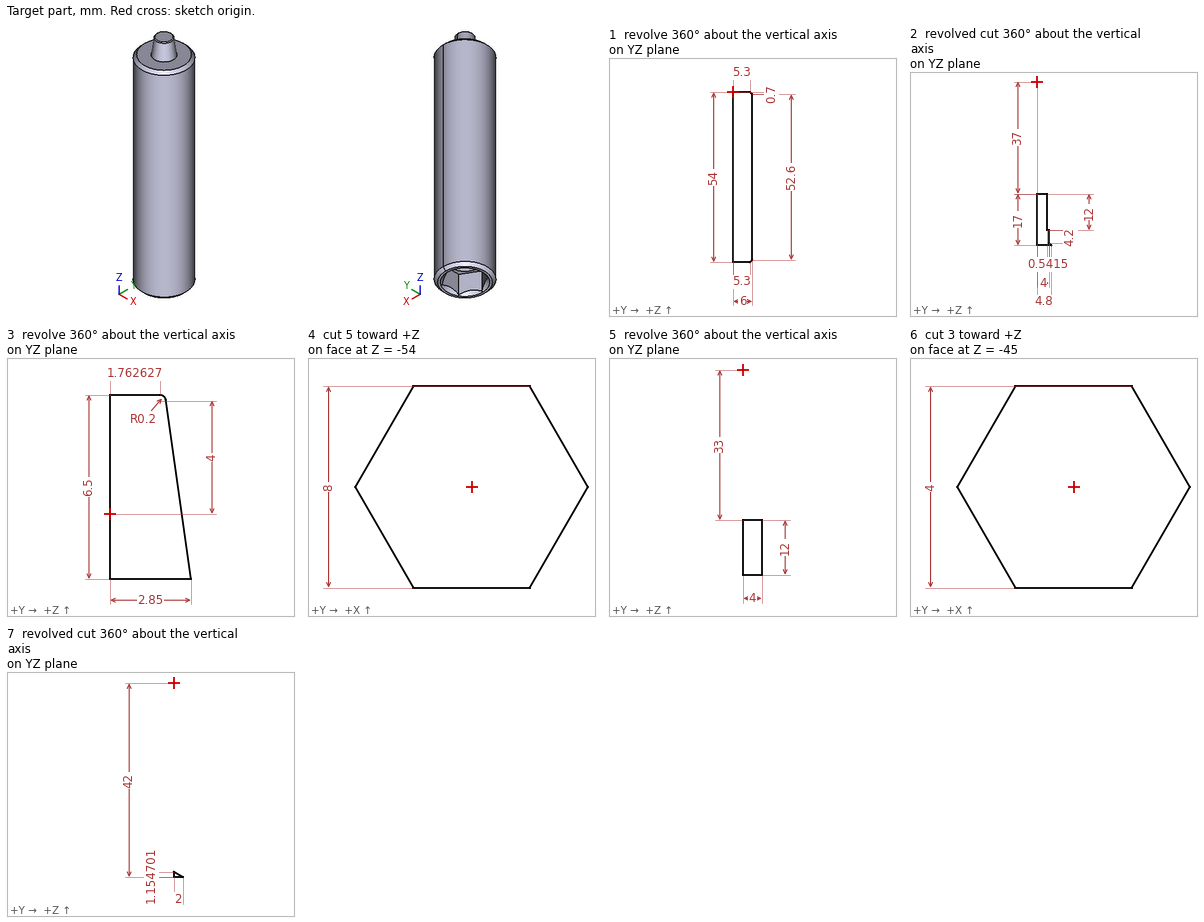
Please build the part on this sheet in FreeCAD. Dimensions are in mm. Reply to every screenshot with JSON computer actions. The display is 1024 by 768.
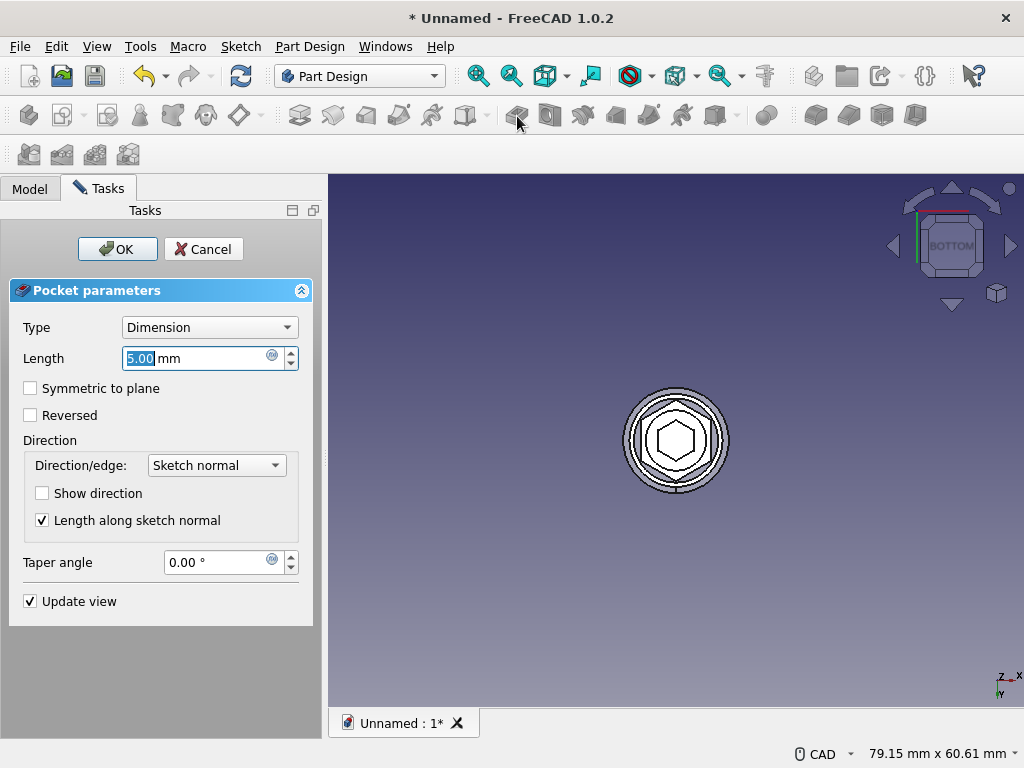
{"action": "type", "text": "3"}
{"action": "key", "text": "Tab"}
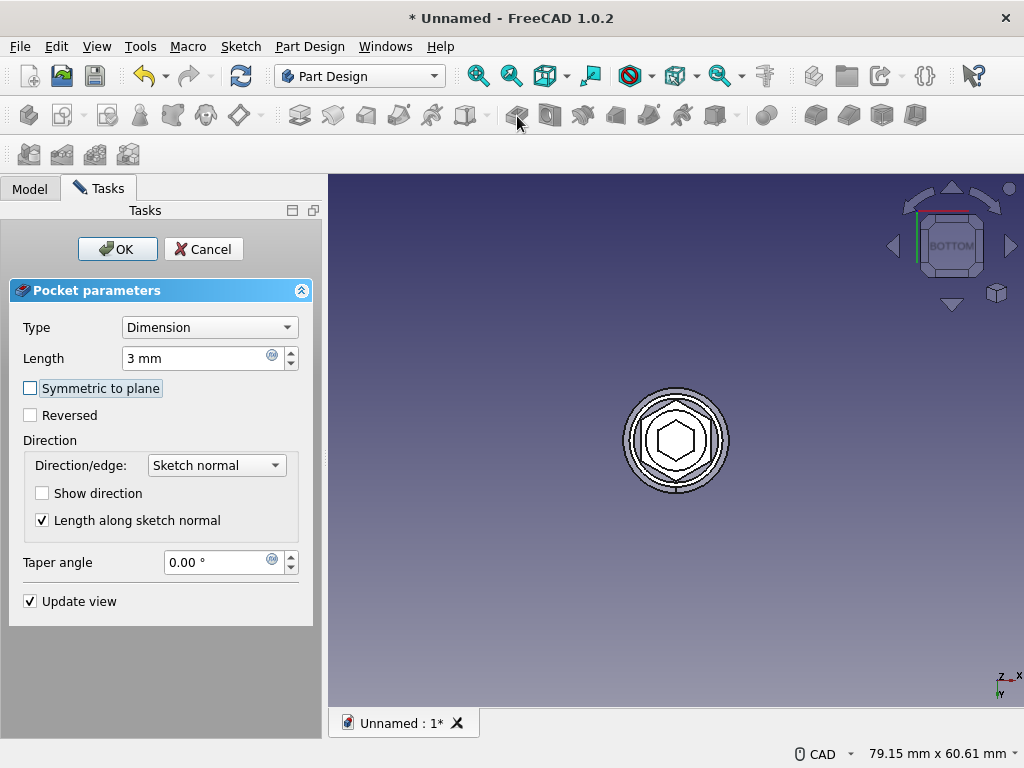
{"action": "left_click", "coordinate": [118, 249]}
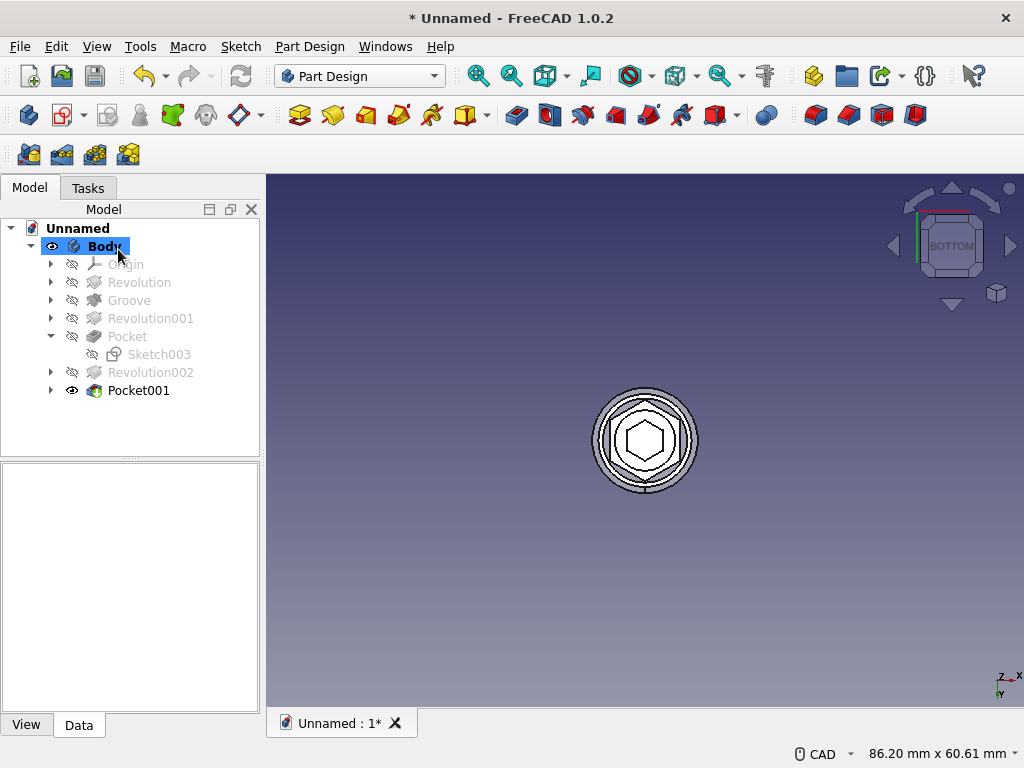
{"action": "left_click", "coordinate": [479, 76]}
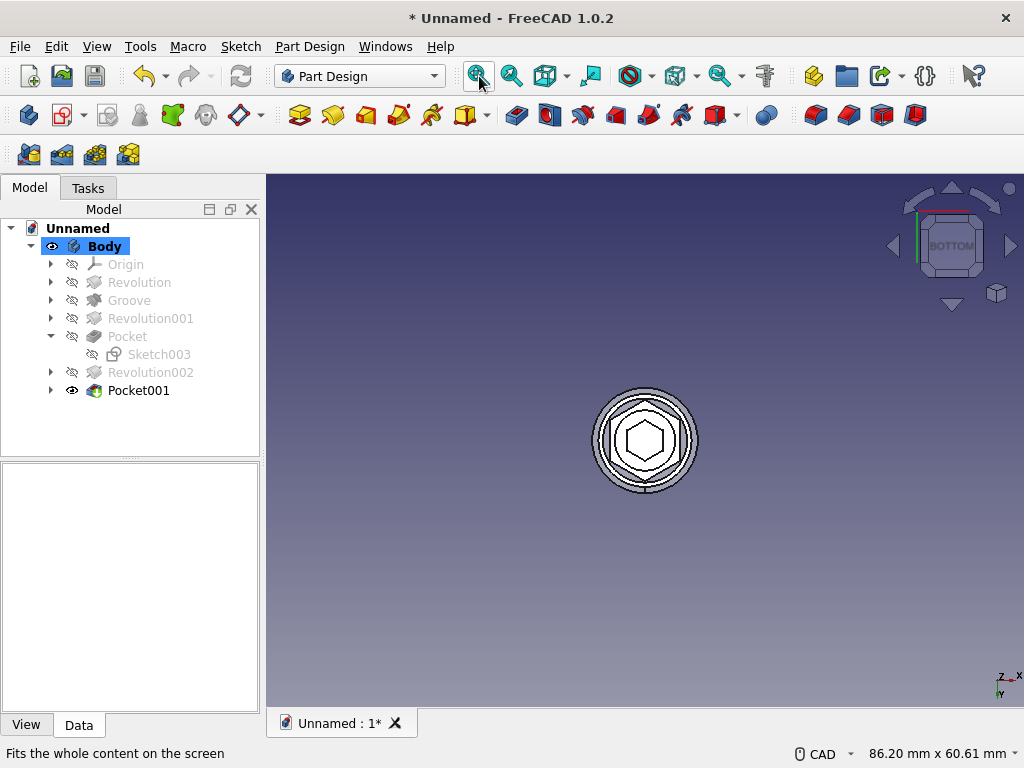
{"action": "left_click", "coordinate": [62, 116]}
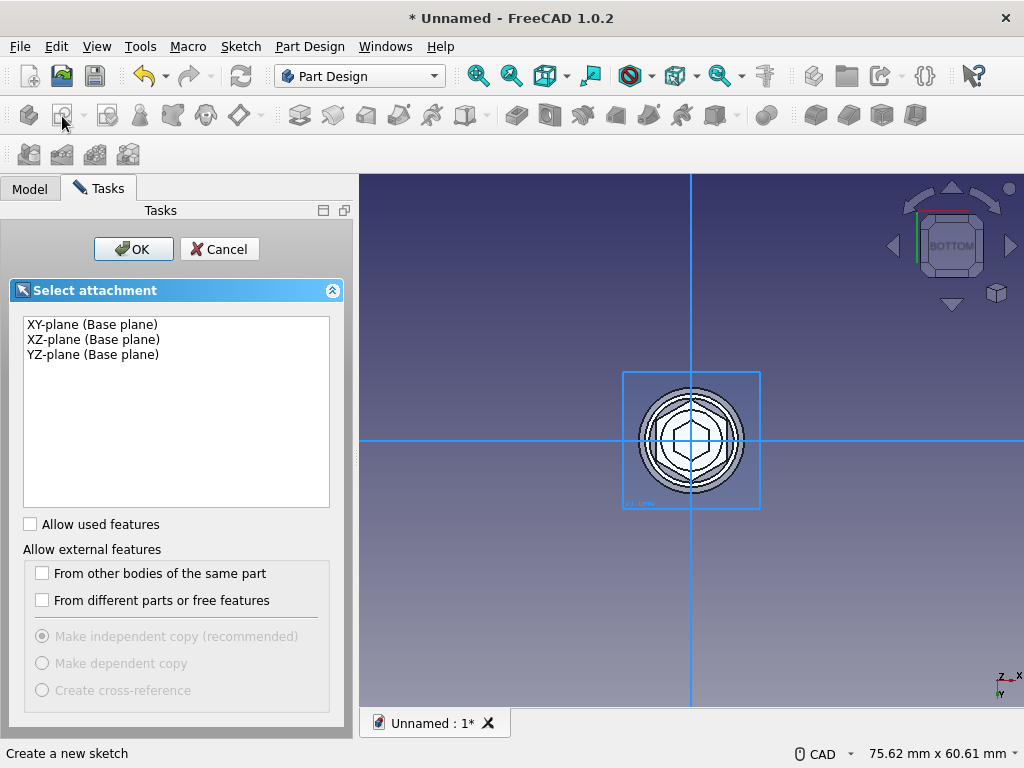
{"action": "left_click", "coordinate": [84, 354]}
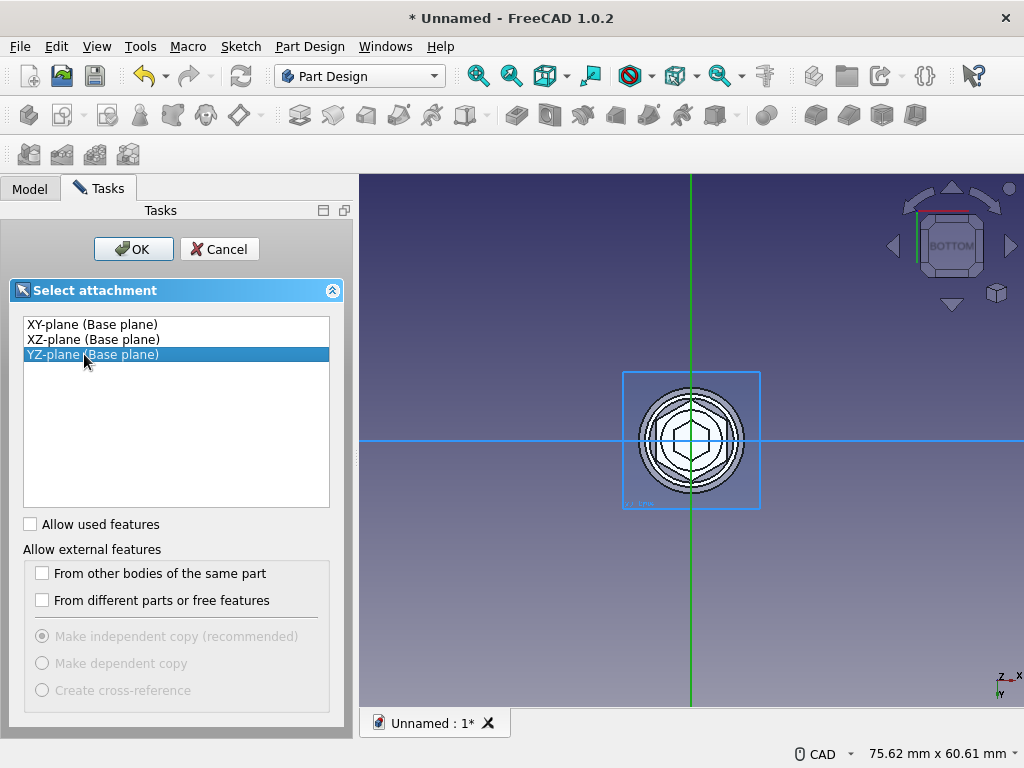
{"action": "left_click", "coordinate": [134, 249]}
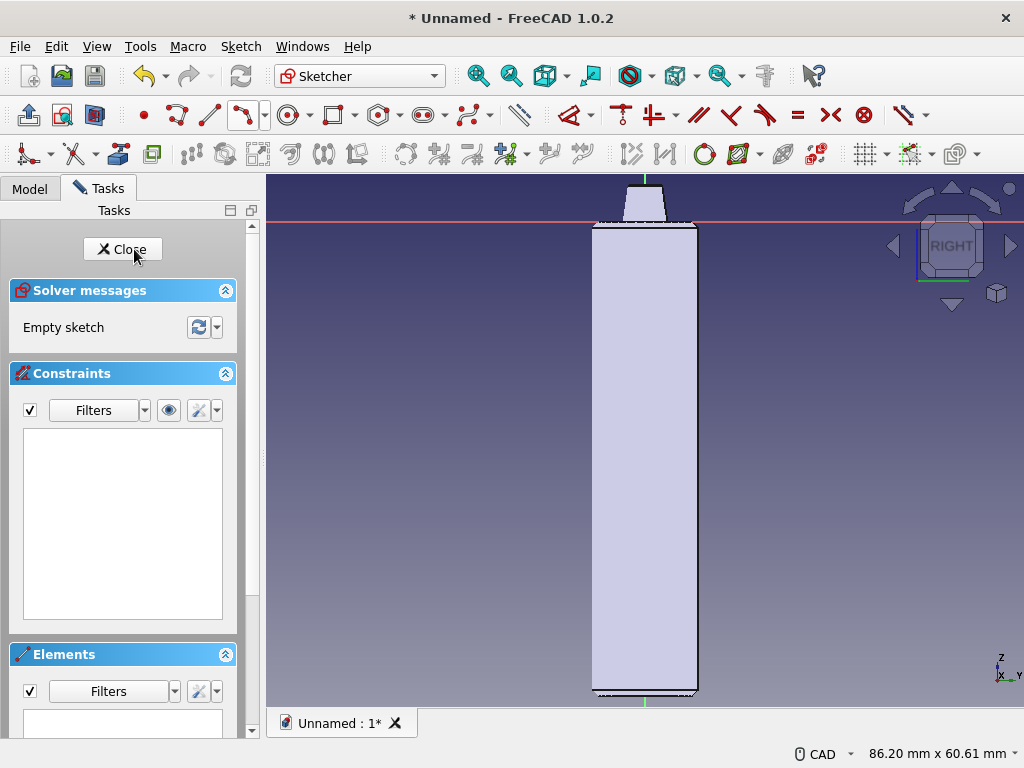
{"action": "left_click", "coordinate": [95, 116]}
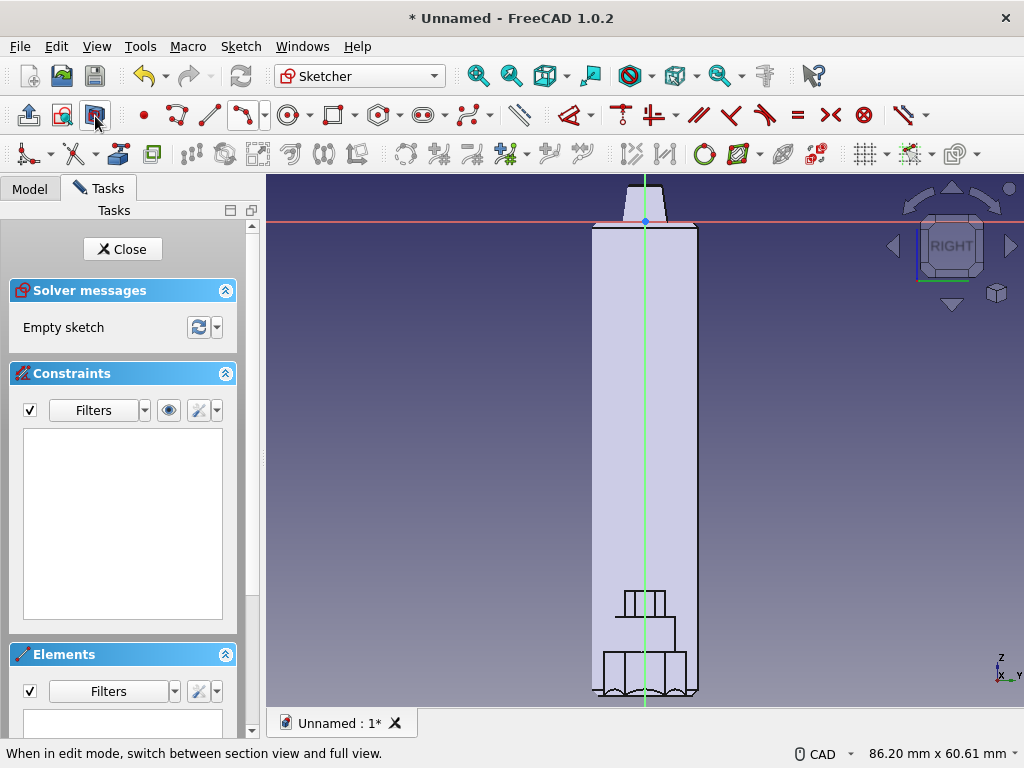
{"action": "scroll", "coordinate": [658, 593], "scroll_direction": "up", "scroll_amount": 15}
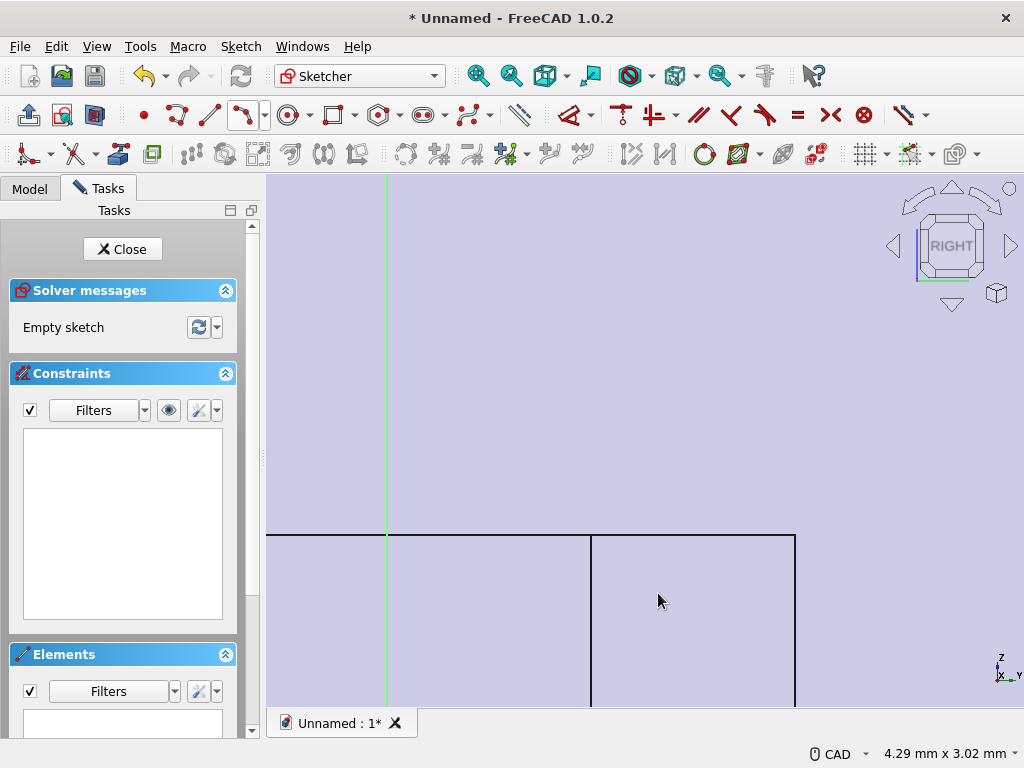
{"action": "left_click", "coordinate": [177, 116]}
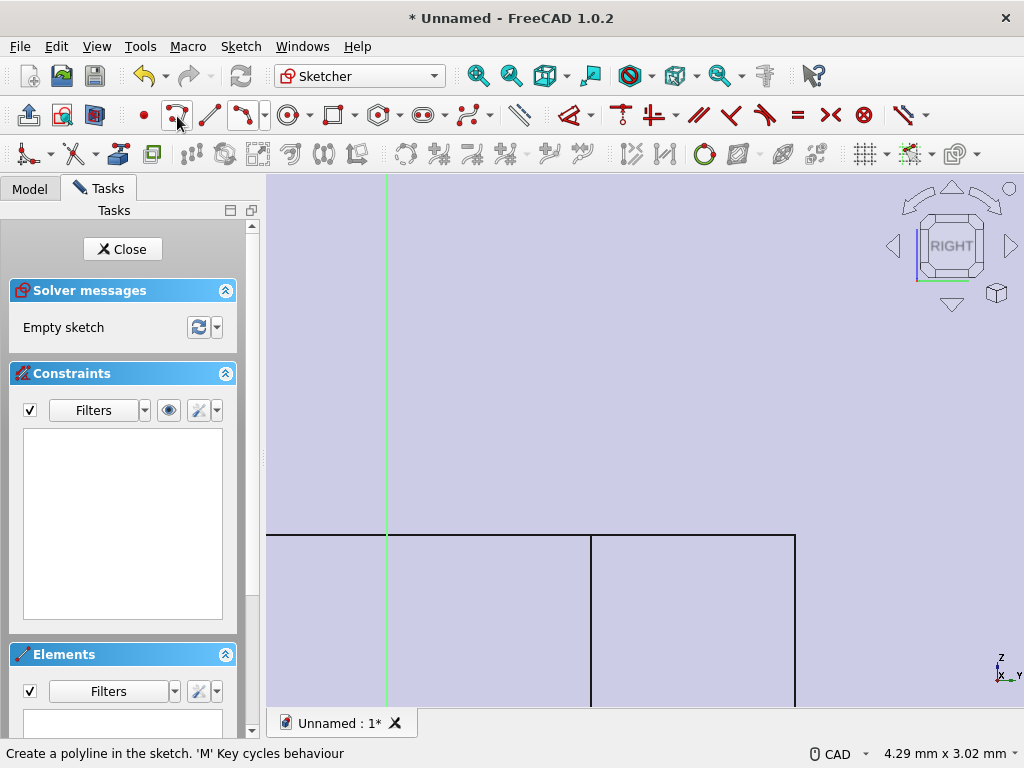
{"action": "left_click", "coordinate": [387, 331]}
{"action": "left_click", "coordinate": [396, 535]}
{"action": "left_click", "coordinate": [740, 535]}
{"action": "left_click", "coordinate": [387, 332]}
{"action": "key", "text": "Escape"}
{"action": "key", "text": "Escape"}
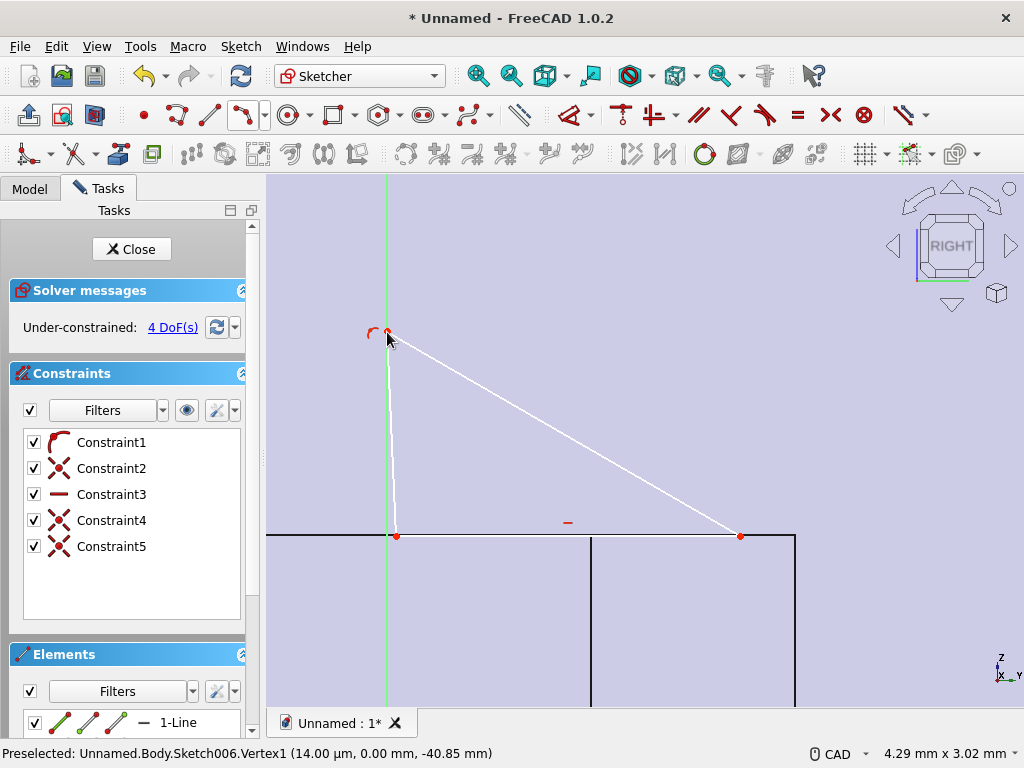
{"action": "left_click", "coordinate": [390, 393]}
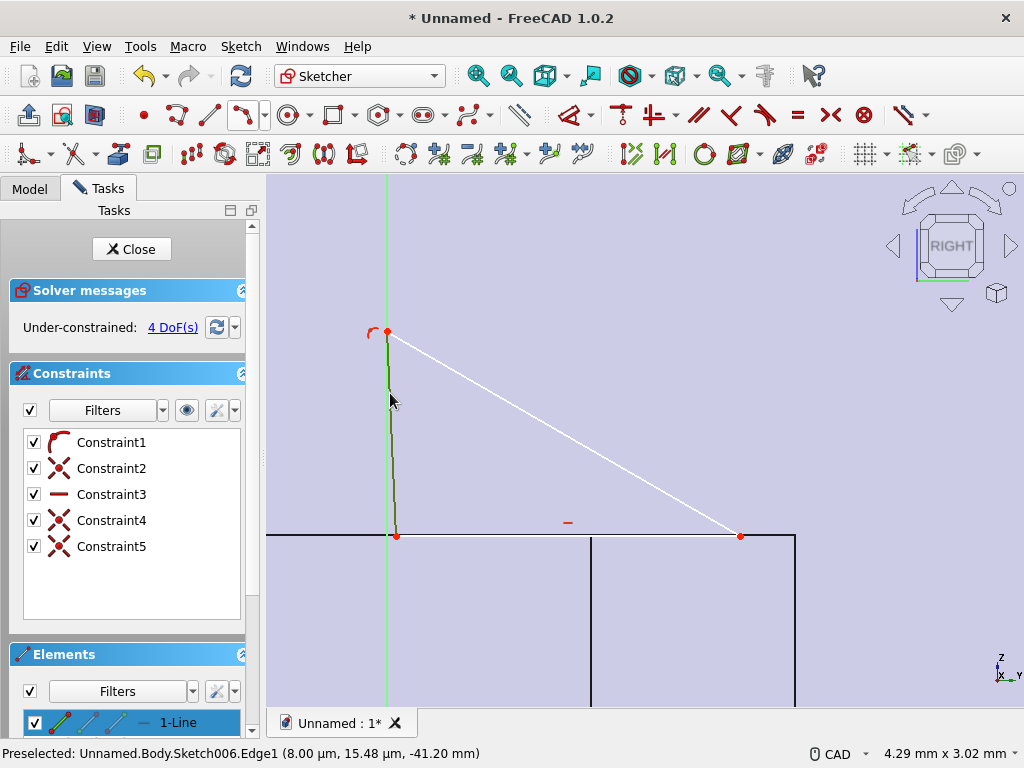
{"action": "key", "text": "v"}